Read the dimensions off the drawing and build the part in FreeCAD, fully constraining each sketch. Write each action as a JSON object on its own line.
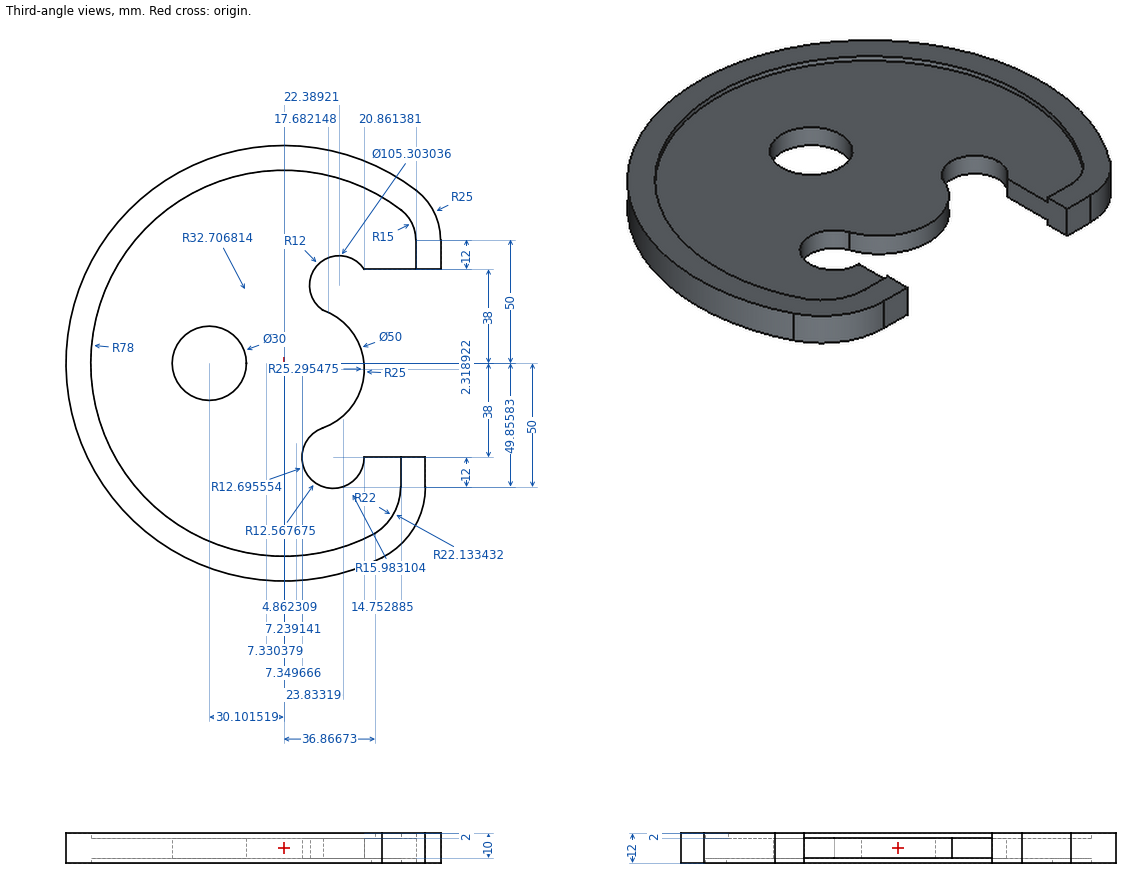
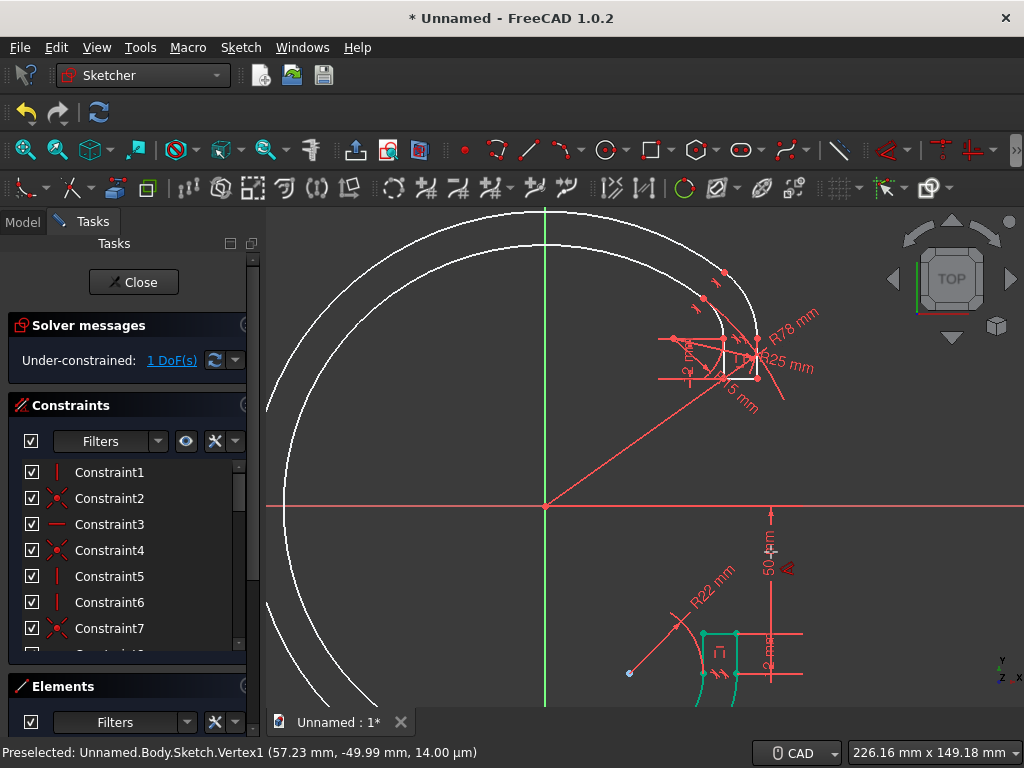
{"action": "left_click", "coordinate": [724, 339]}
{"action": "left_click", "coordinate": [758, 423]}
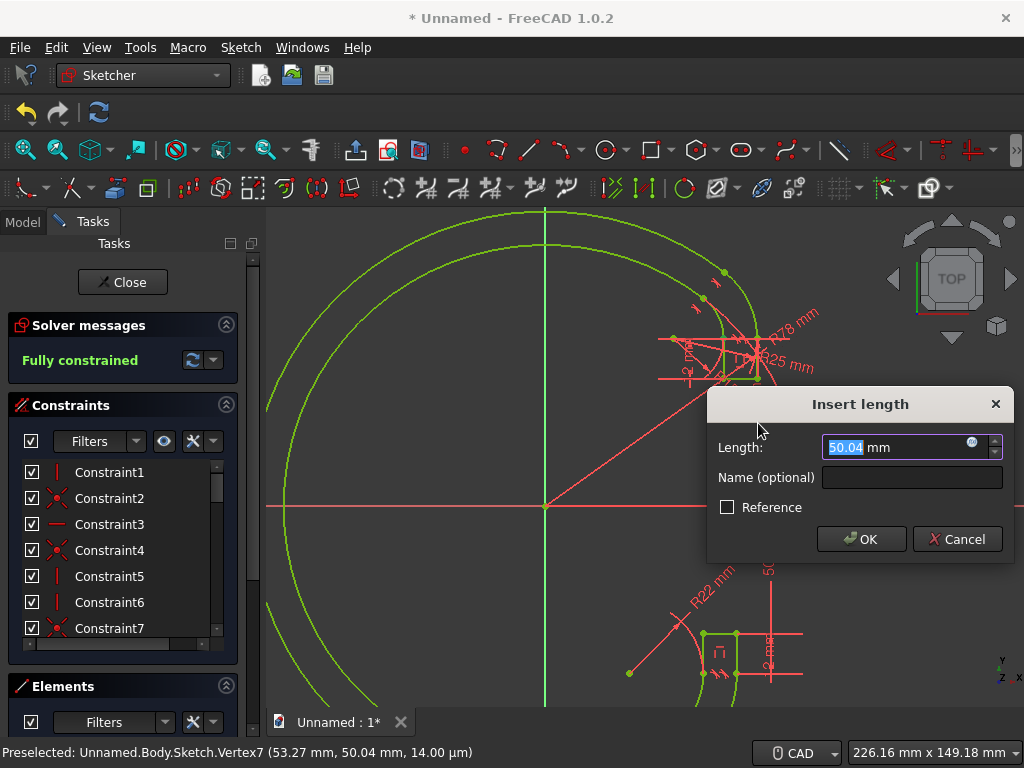
{"action": "type", "text": "50"}
{"action": "key", "text": "Return"}
{"action": "key", "text": "Escape"}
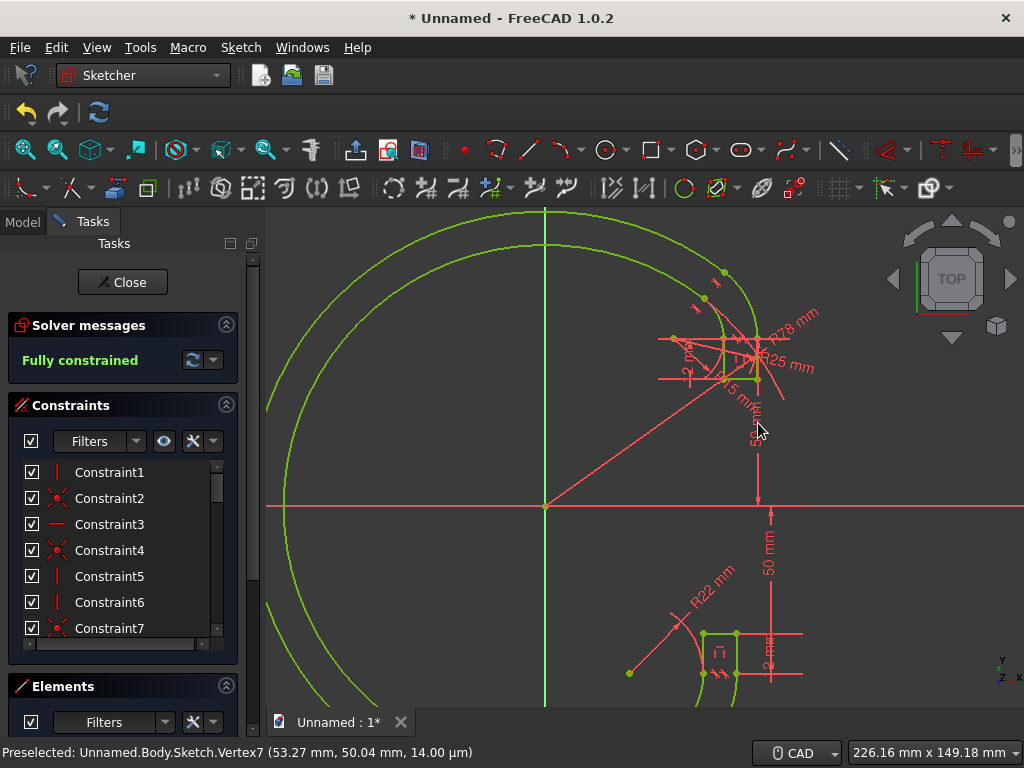
{"action": "left_click", "coordinate": [123, 282]}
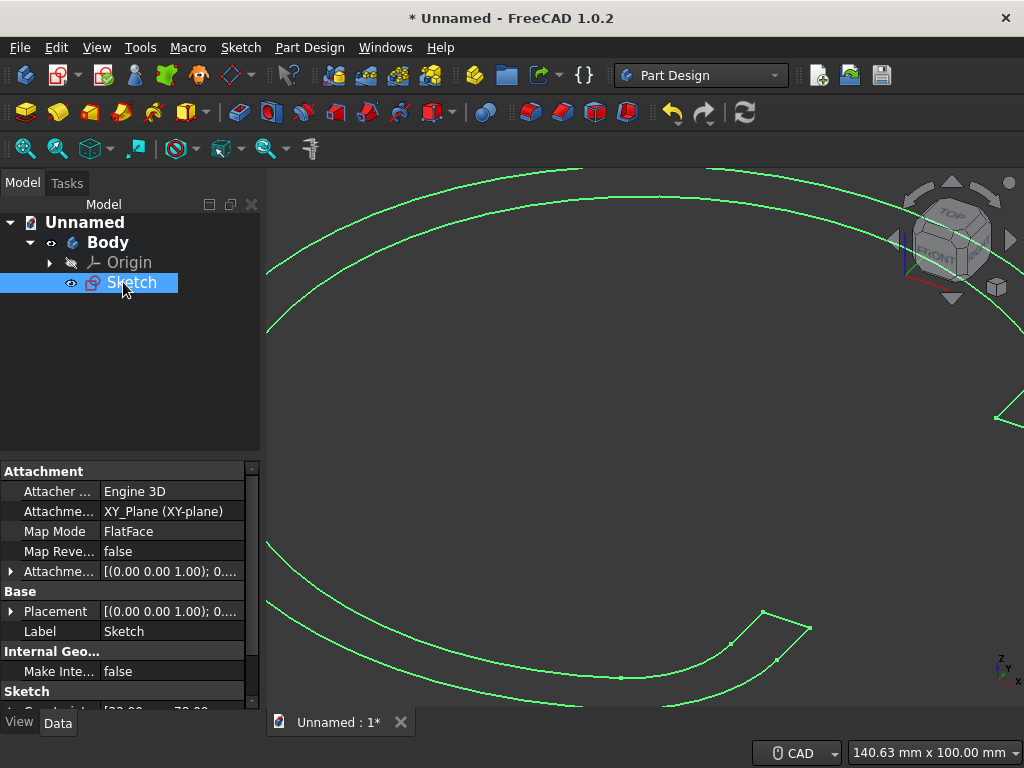
{"action": "left_click", "coordinate": [26, 112]}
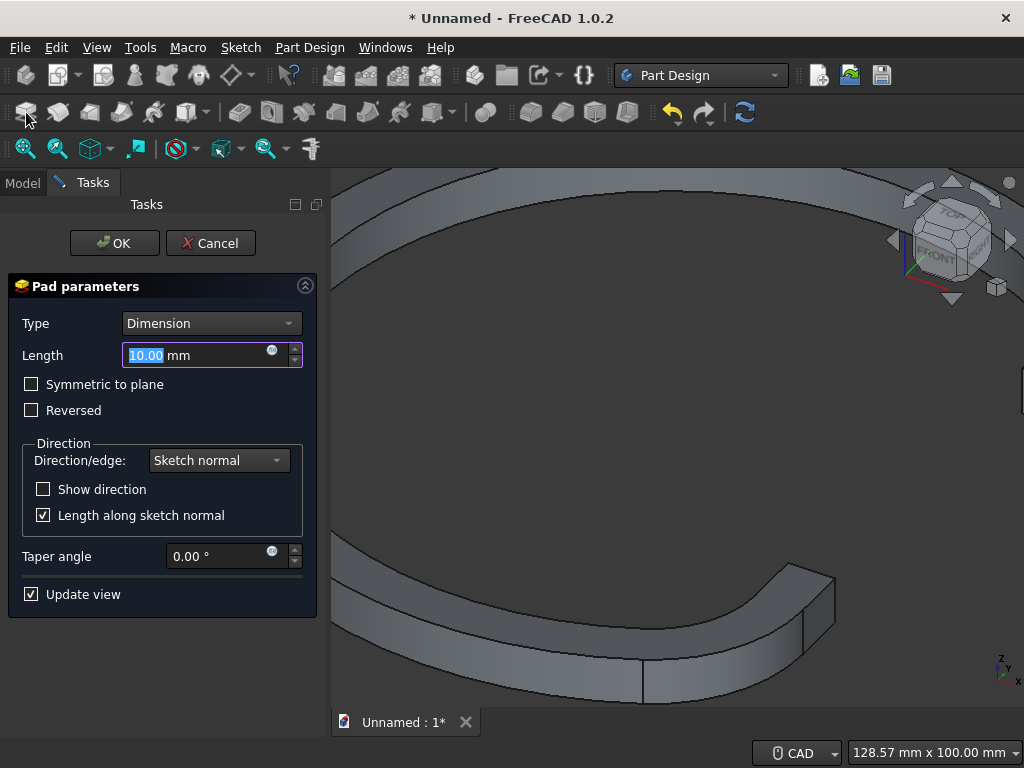
{"action": "type", "text": "12"}
{"action": "key", "text": "Tab"}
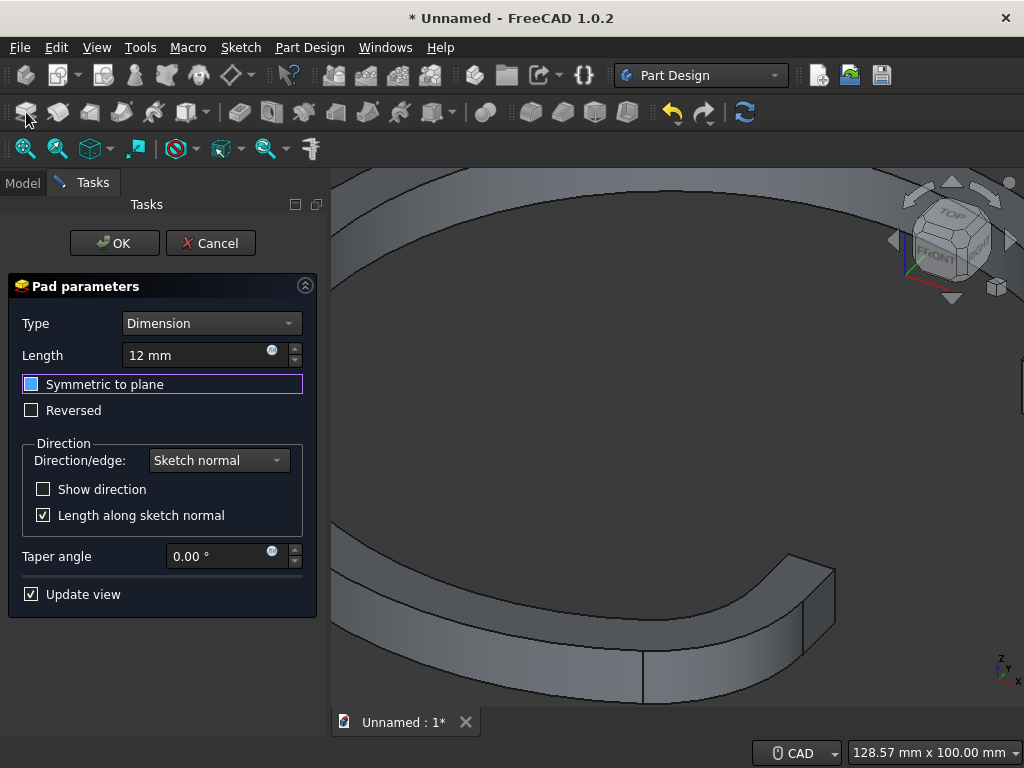
{"action": "left_click", "coordinate": [30, 384]}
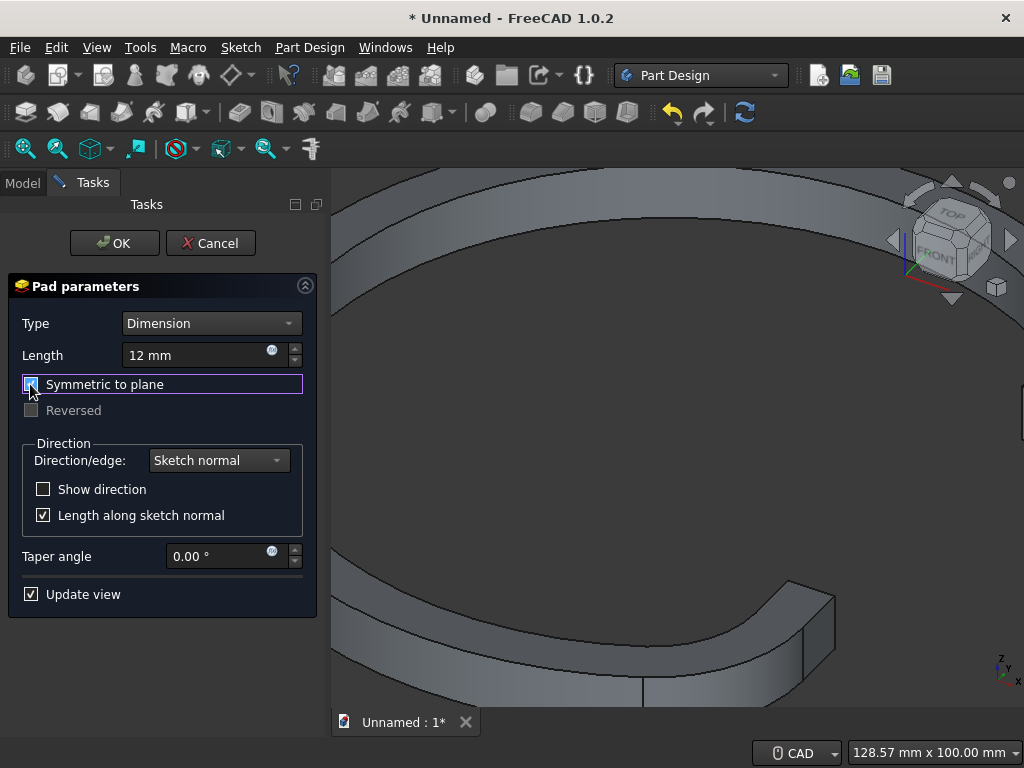
{"action": "left_click", "coordinate": [115, 243]}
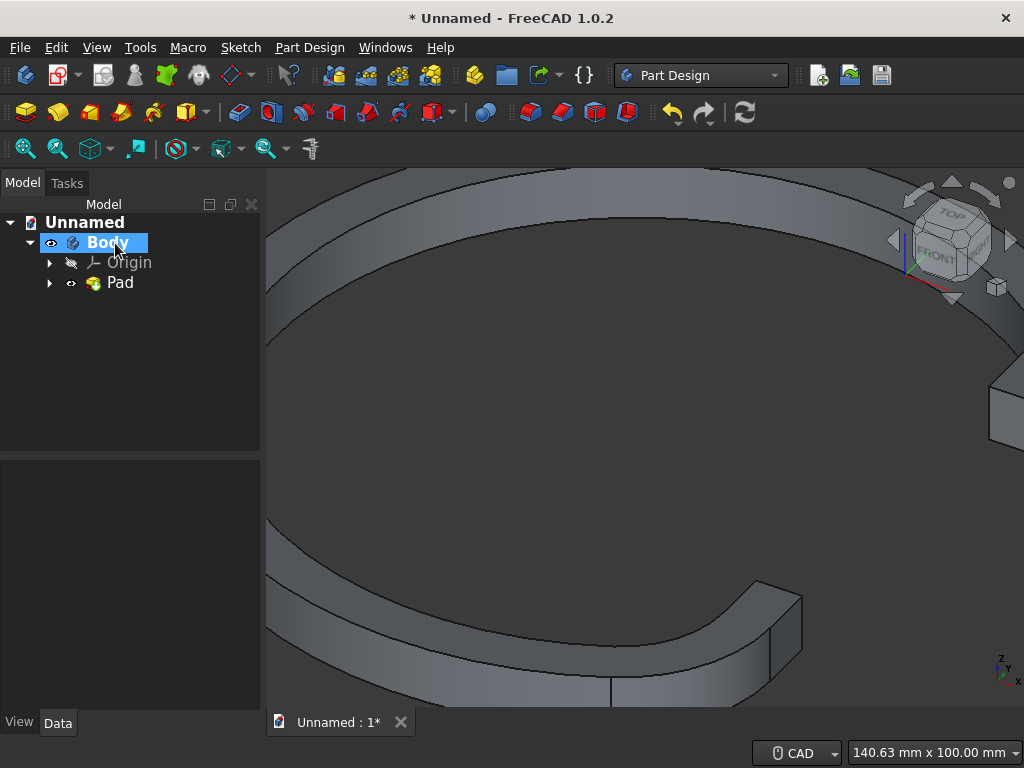
{"action": "key", "text": "v f"}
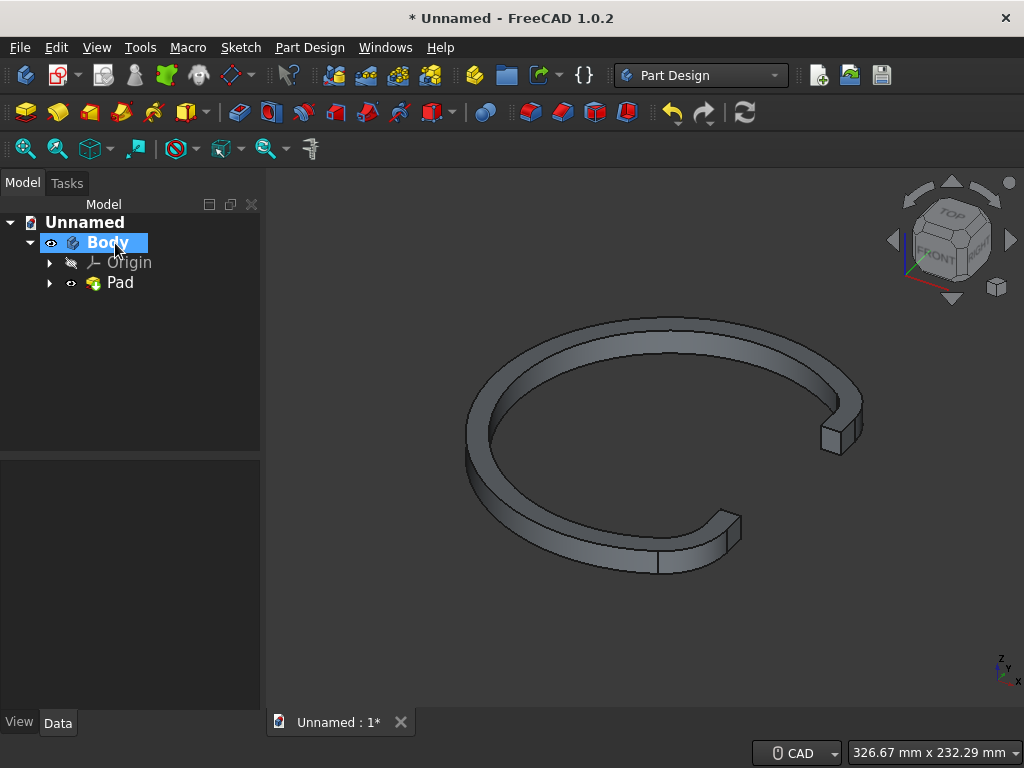
{"action": "left_click", "coordinate": [644, 541]}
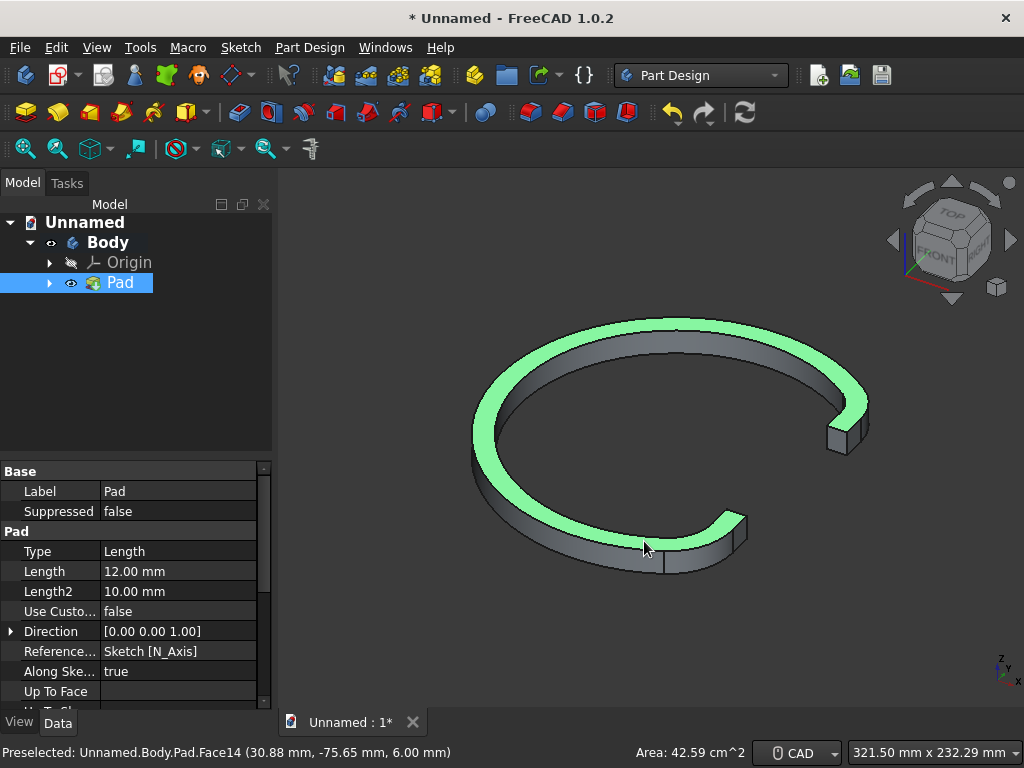
{"action": "left_click", "coordinate": [58, 76]}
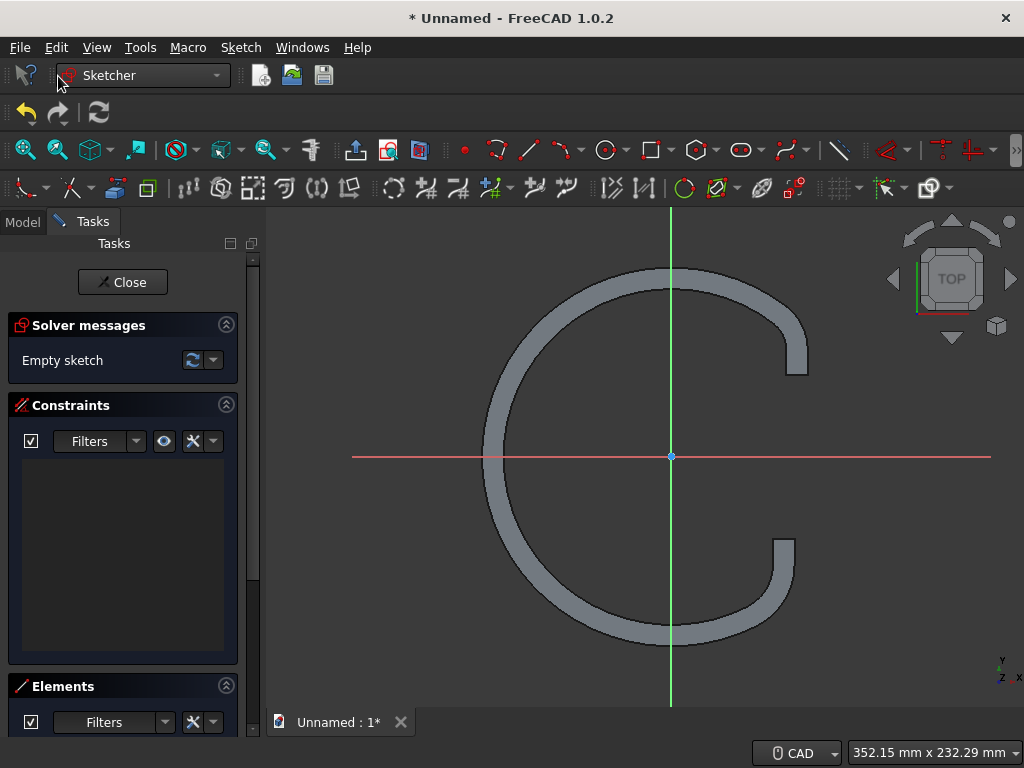
{"action": "key", "text": "g m"}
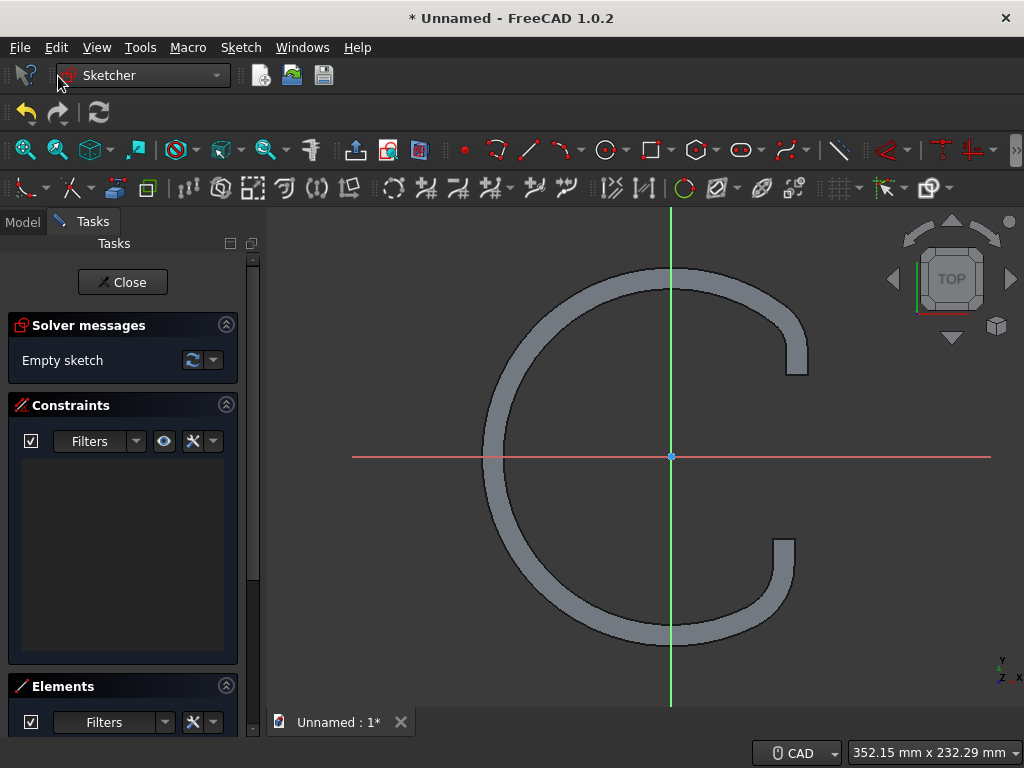
{"action": "left_click", "coordinate": [741, 375]}
{"action": "left_click", "coordinate": [786, 375]}
{"action": "left_click", "coordinate": [786, 349]}
{"action": "right_click", "coordinate": [786, 349]}